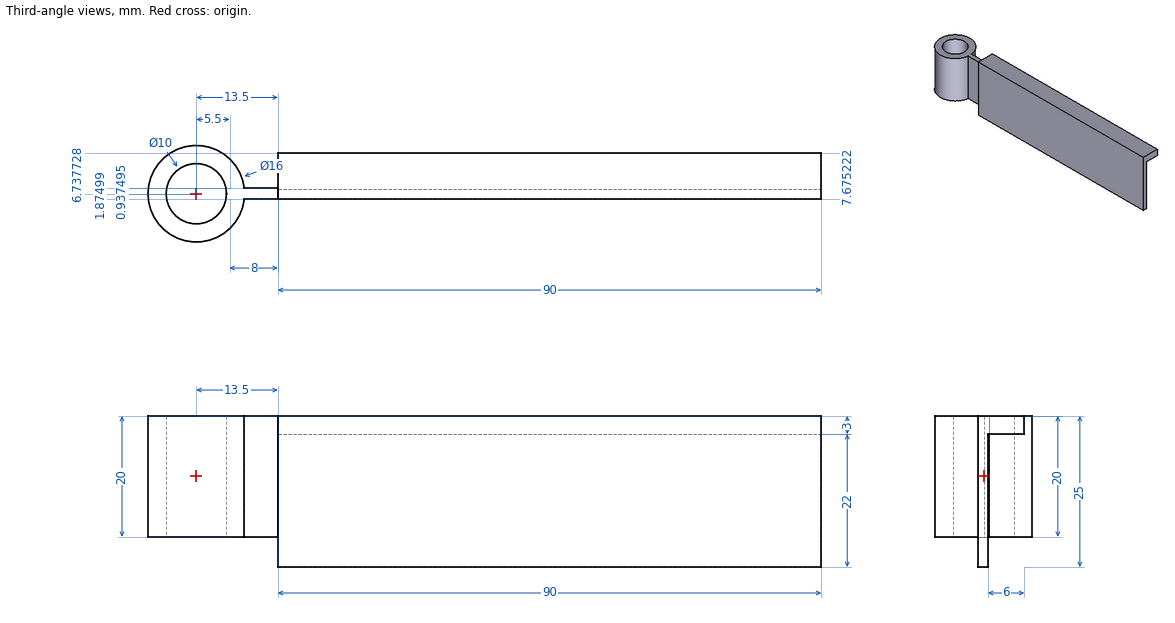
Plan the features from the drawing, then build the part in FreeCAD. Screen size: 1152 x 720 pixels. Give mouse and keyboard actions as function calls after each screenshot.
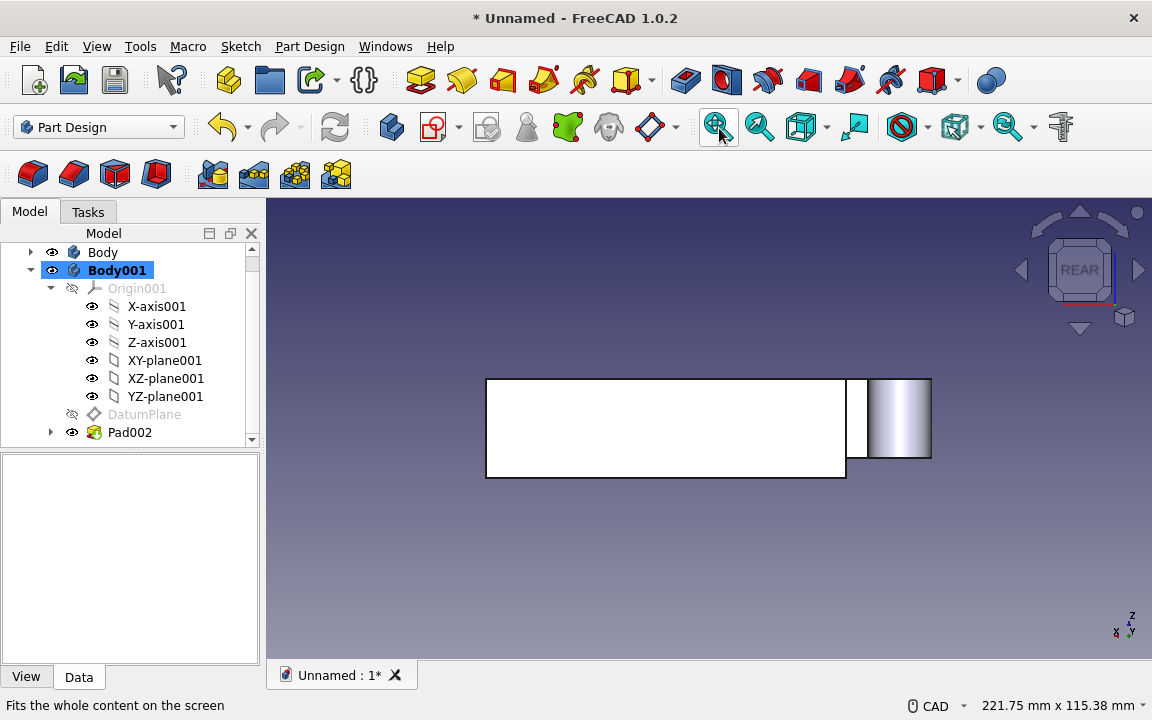
click(719, 128)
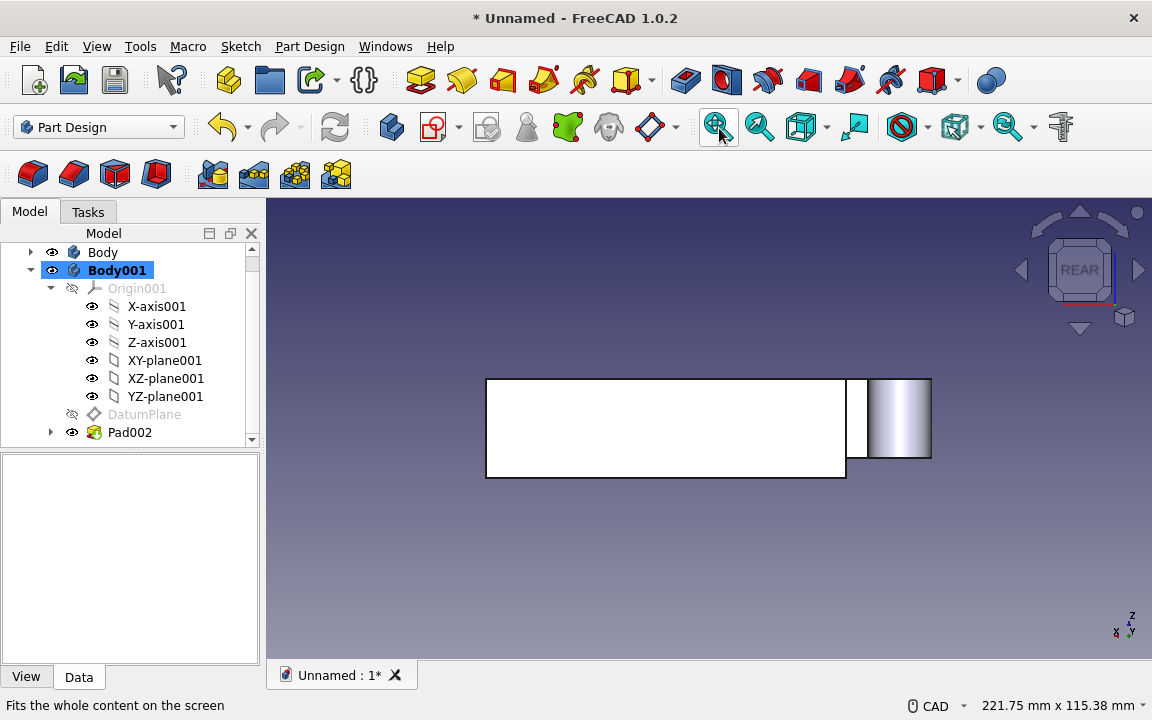
click(563, 428)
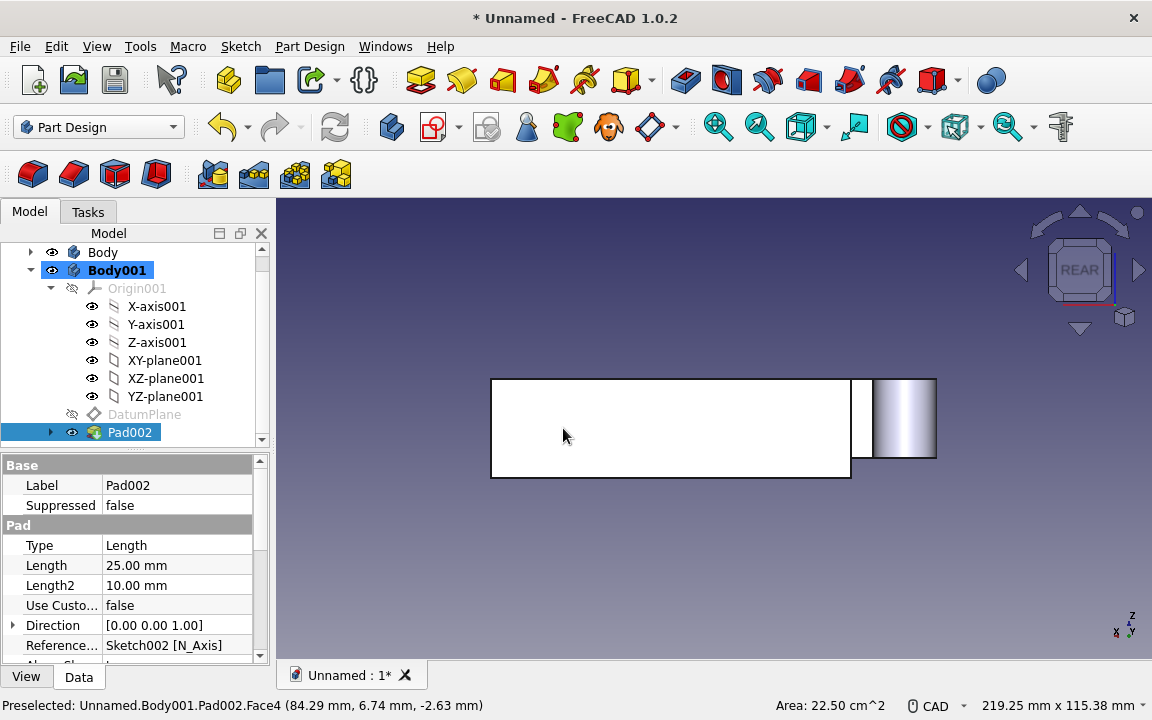
click(432, 128)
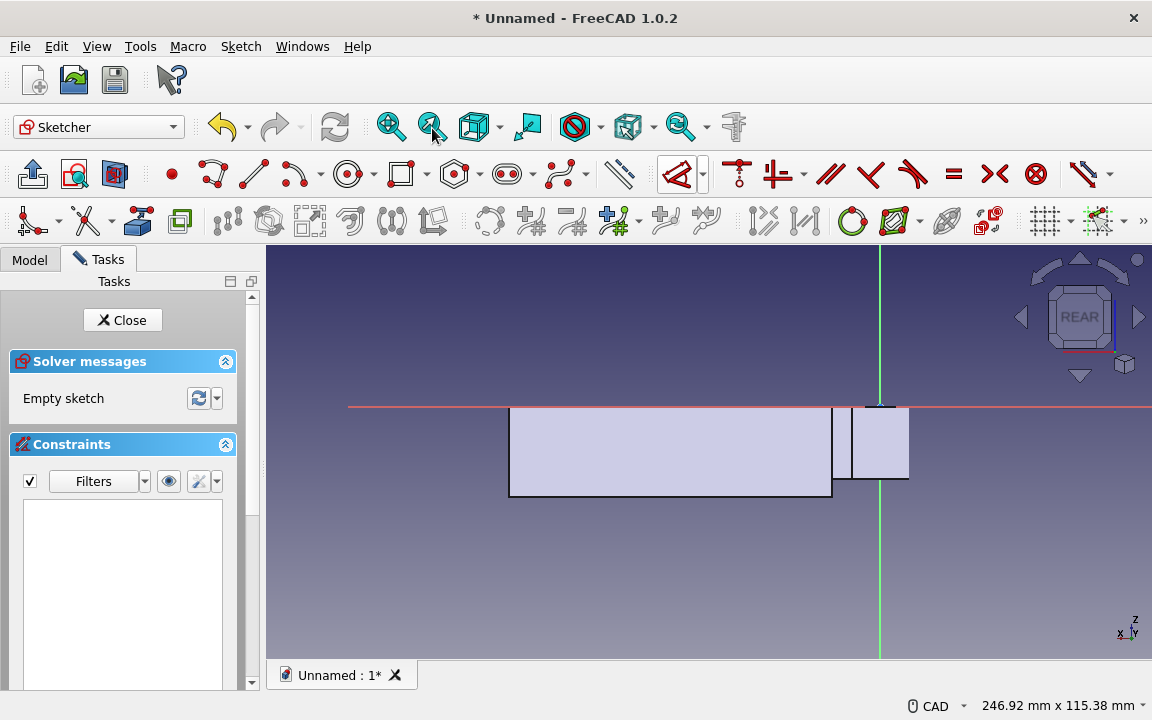
click(400, 174)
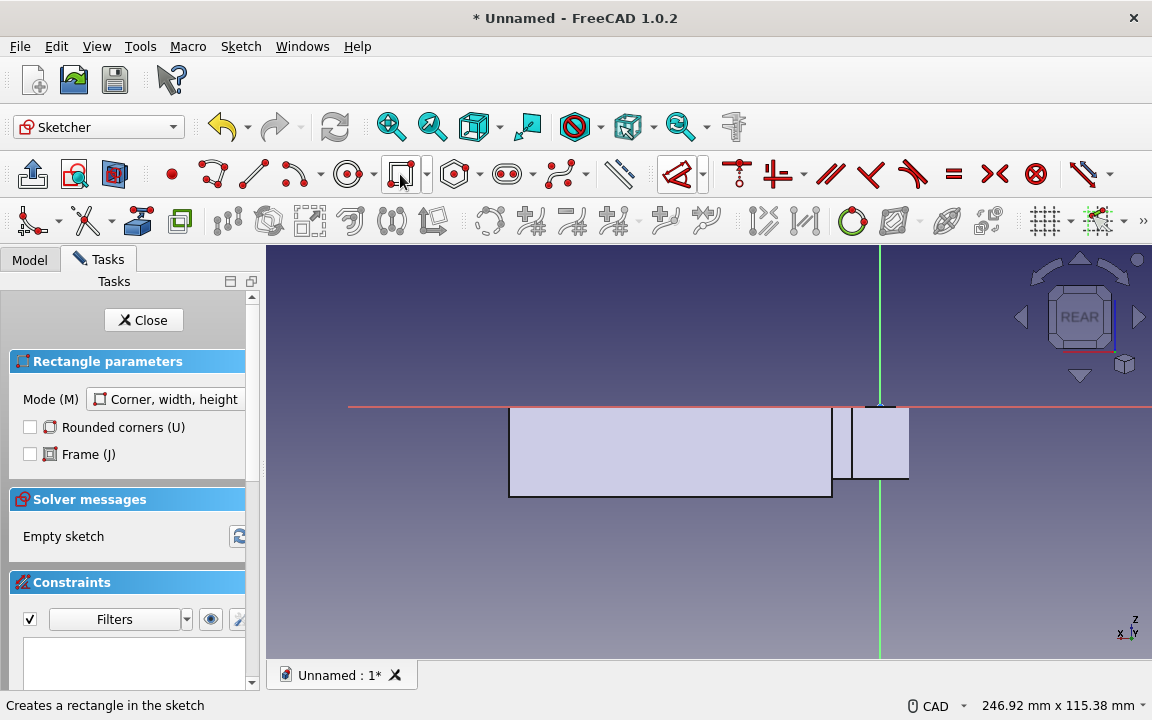
scroll(509, 418, up, 2)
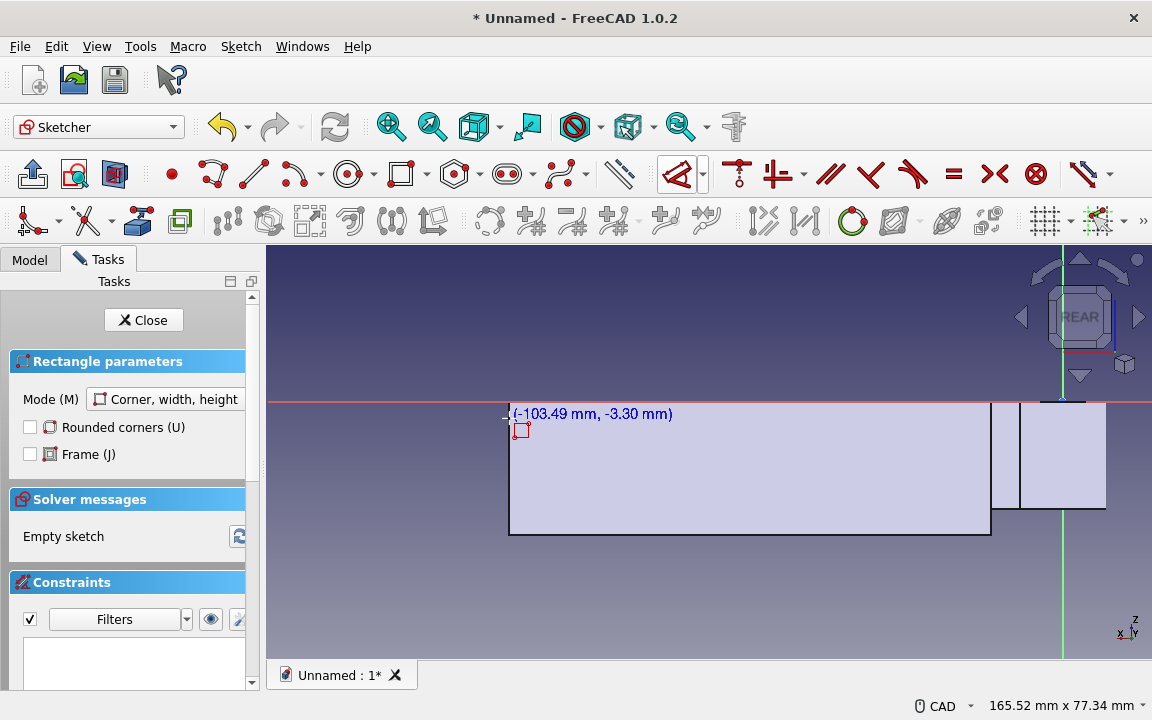
click(509, 418)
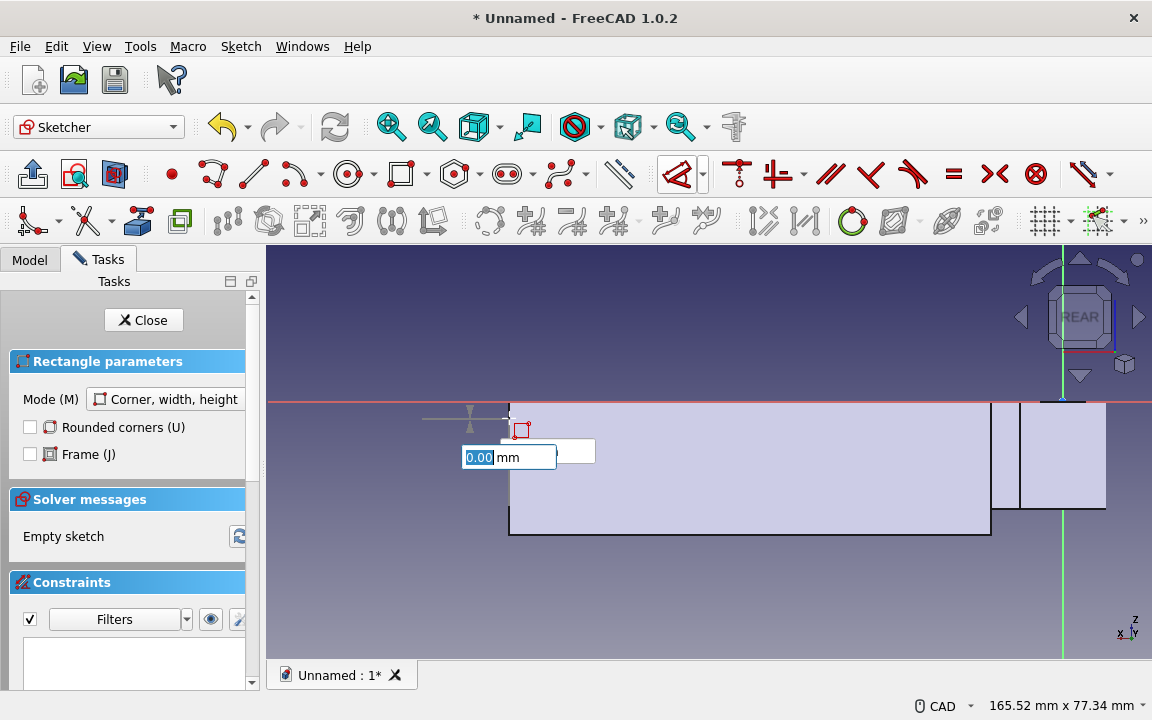
scroll(294, 377, down, 1)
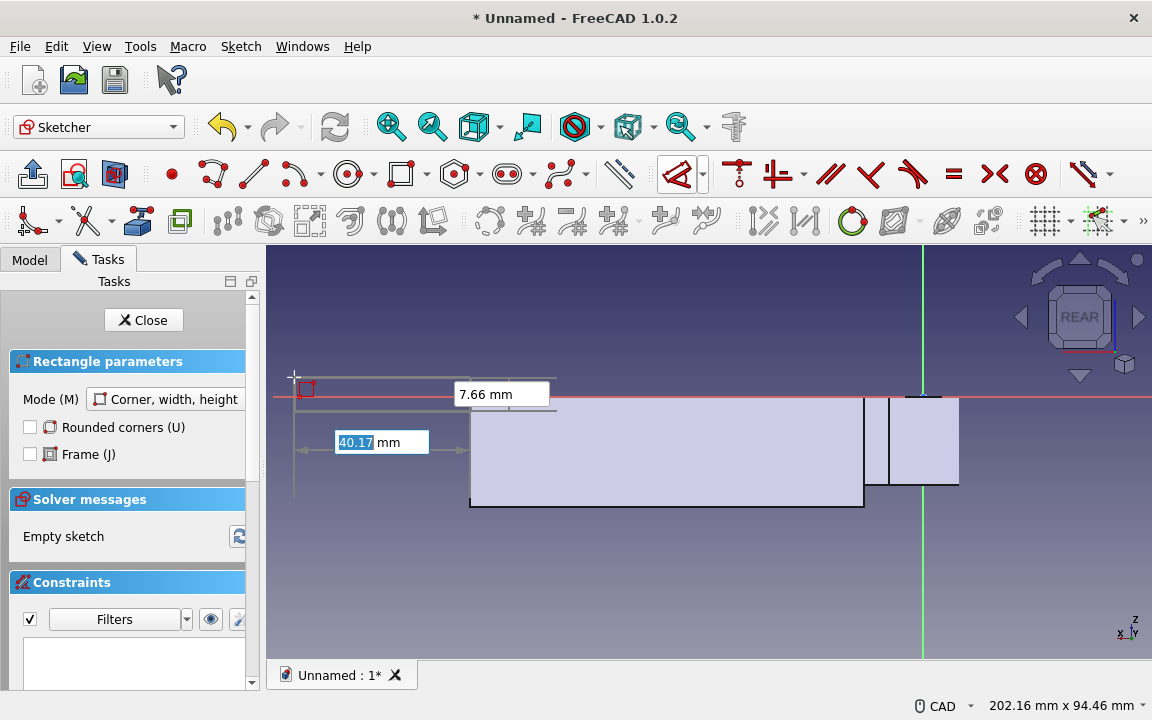
click(864, 507)
key(Escape)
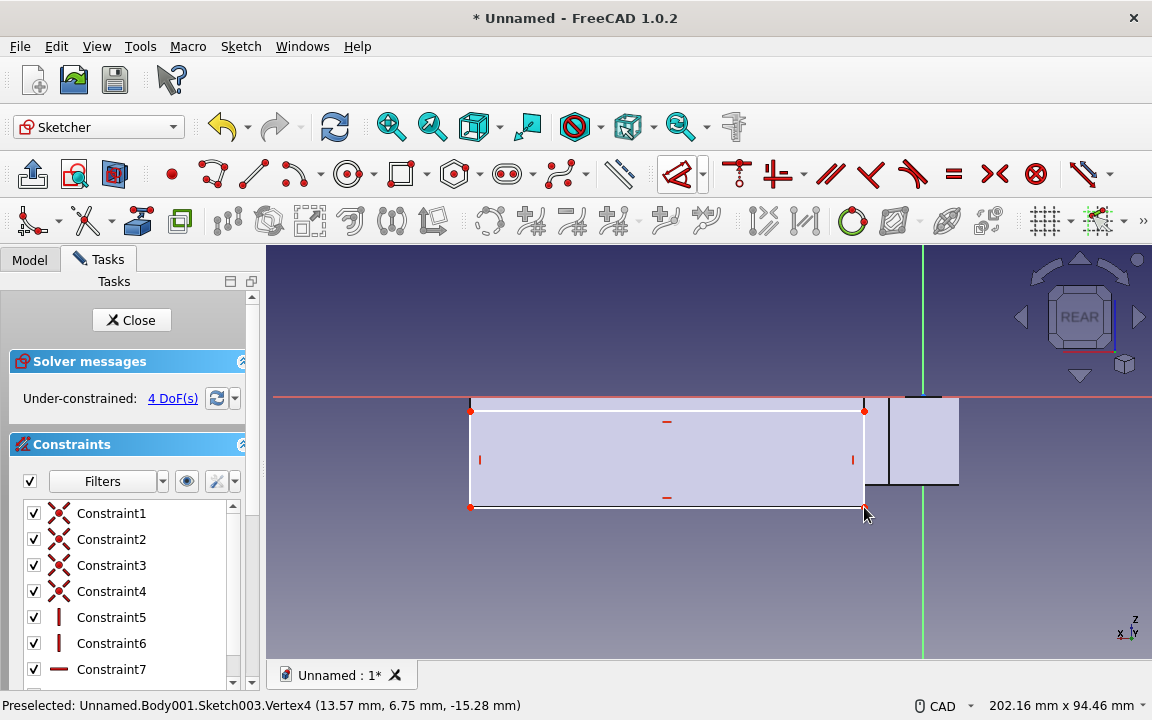
click(470, 440)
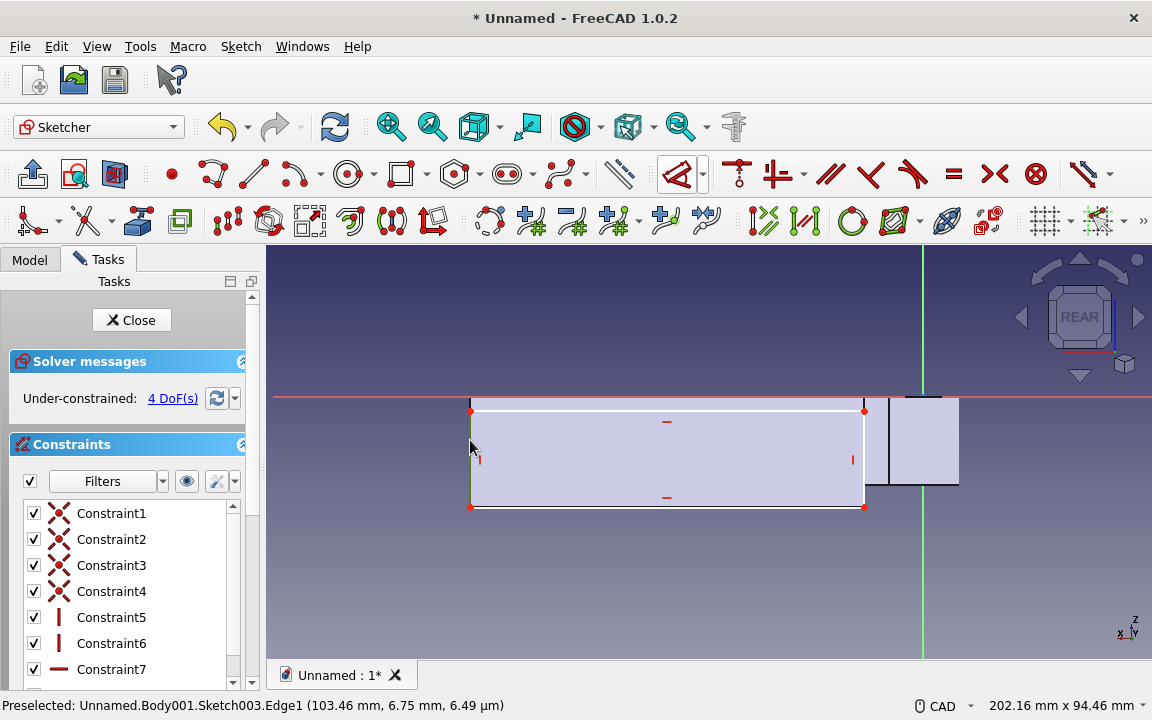
key(i)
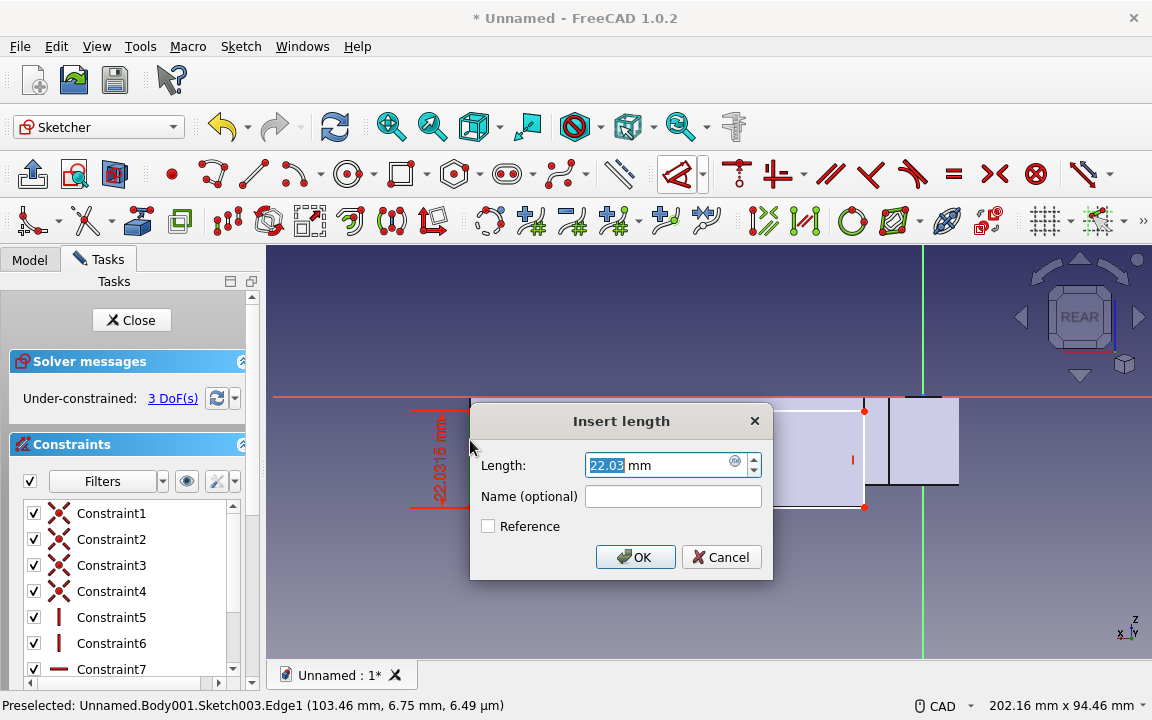
text(22)
key(Return)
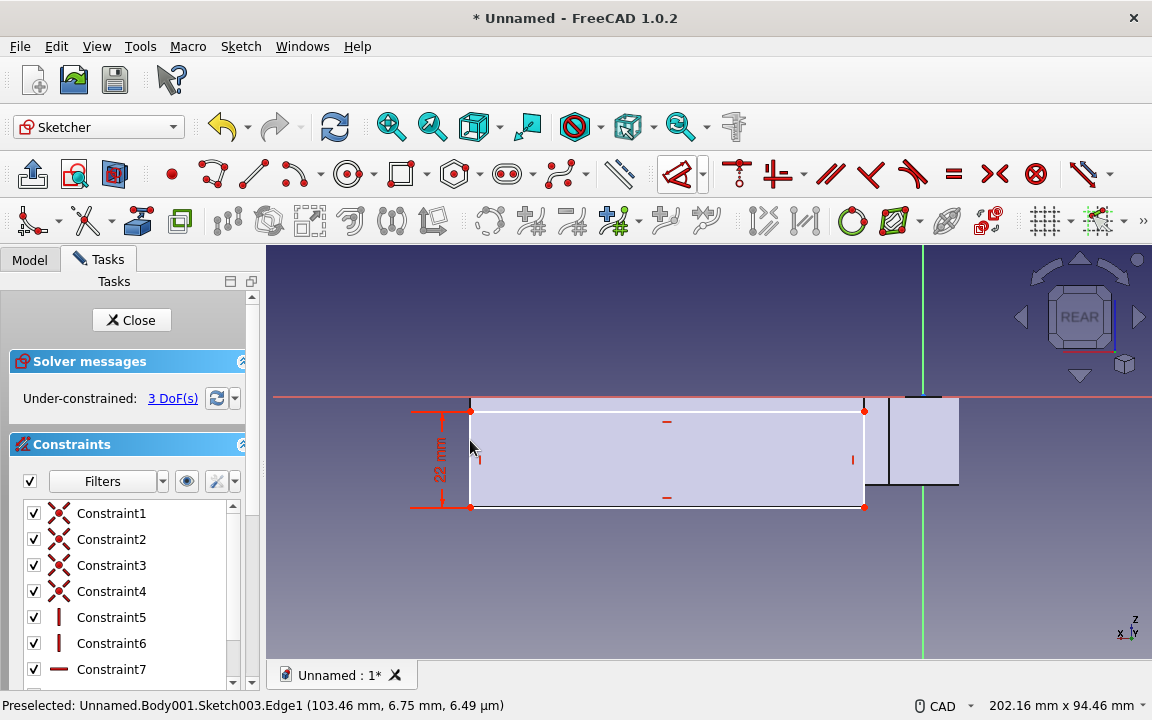
click(588, 508)